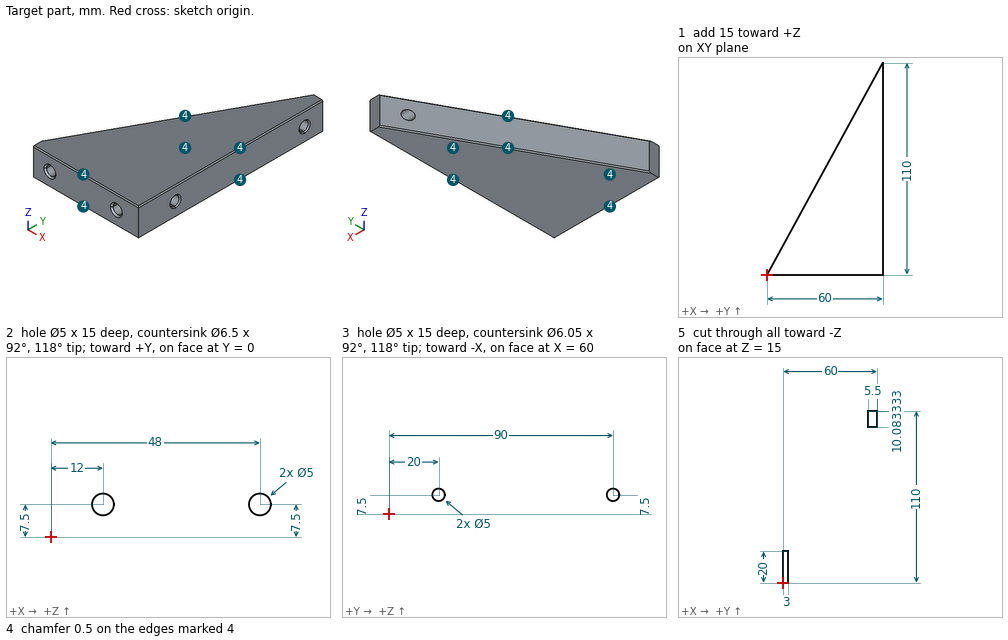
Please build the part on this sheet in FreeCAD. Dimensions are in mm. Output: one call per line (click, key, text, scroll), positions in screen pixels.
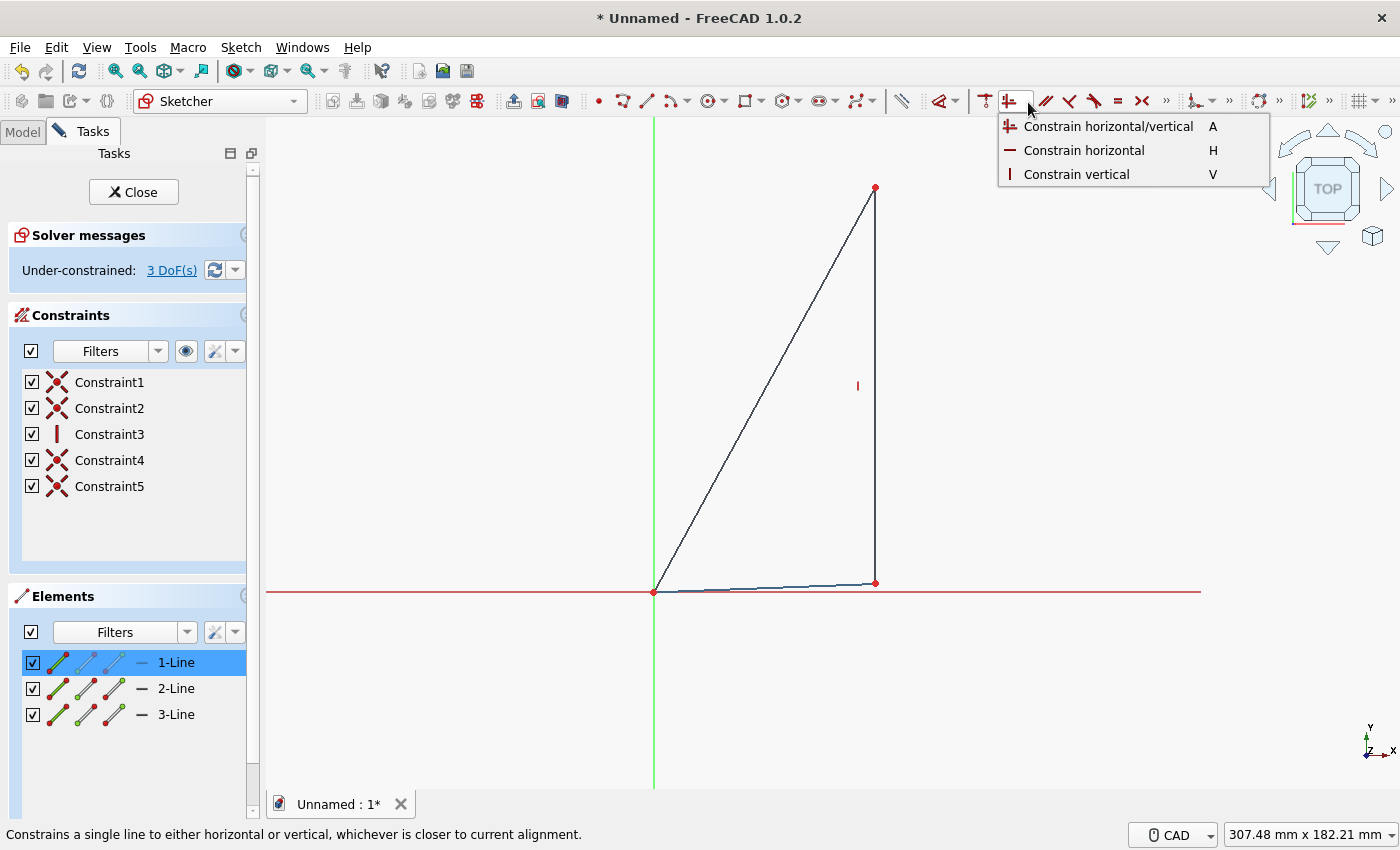
click(1134, 150)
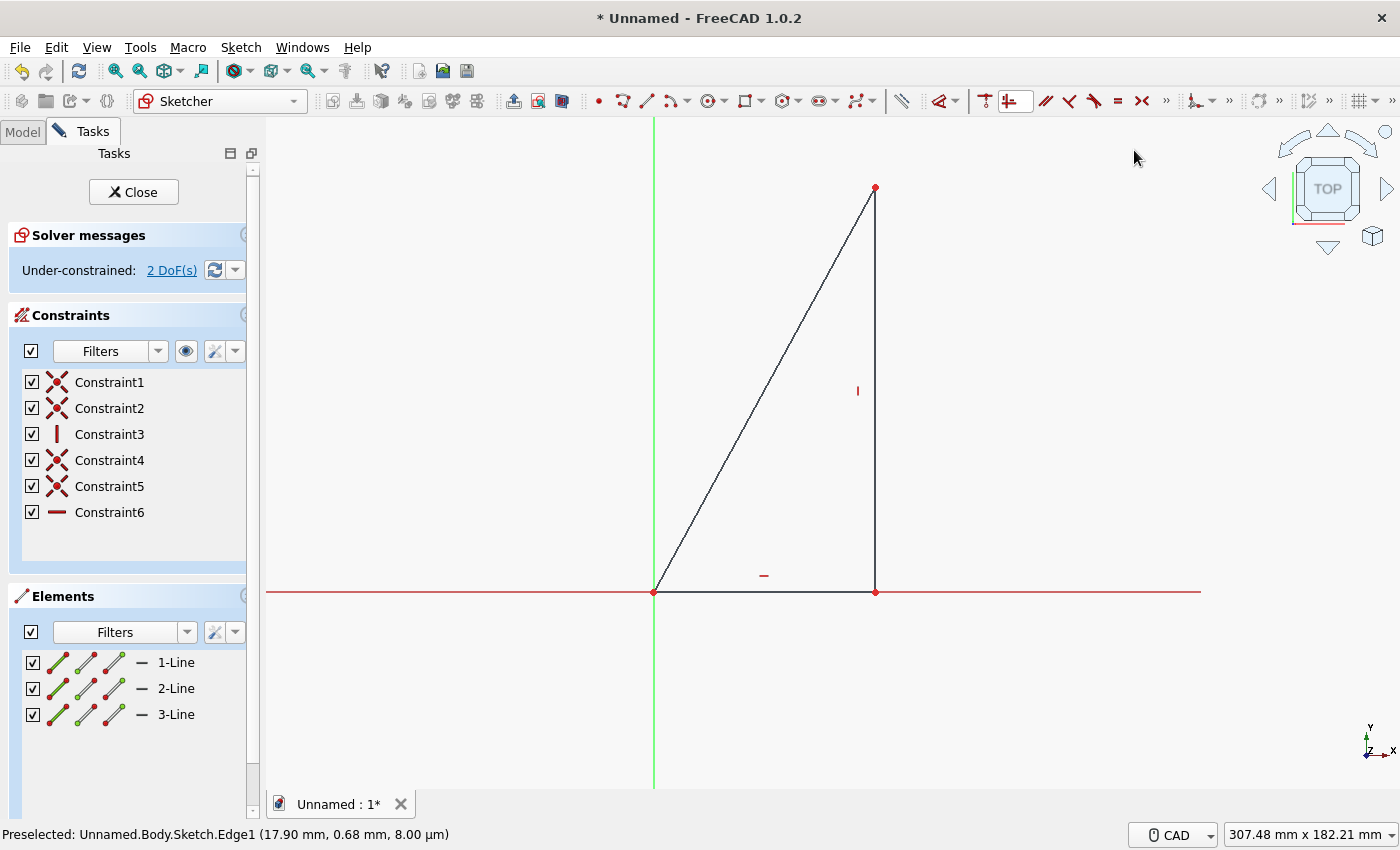
click(940, 102)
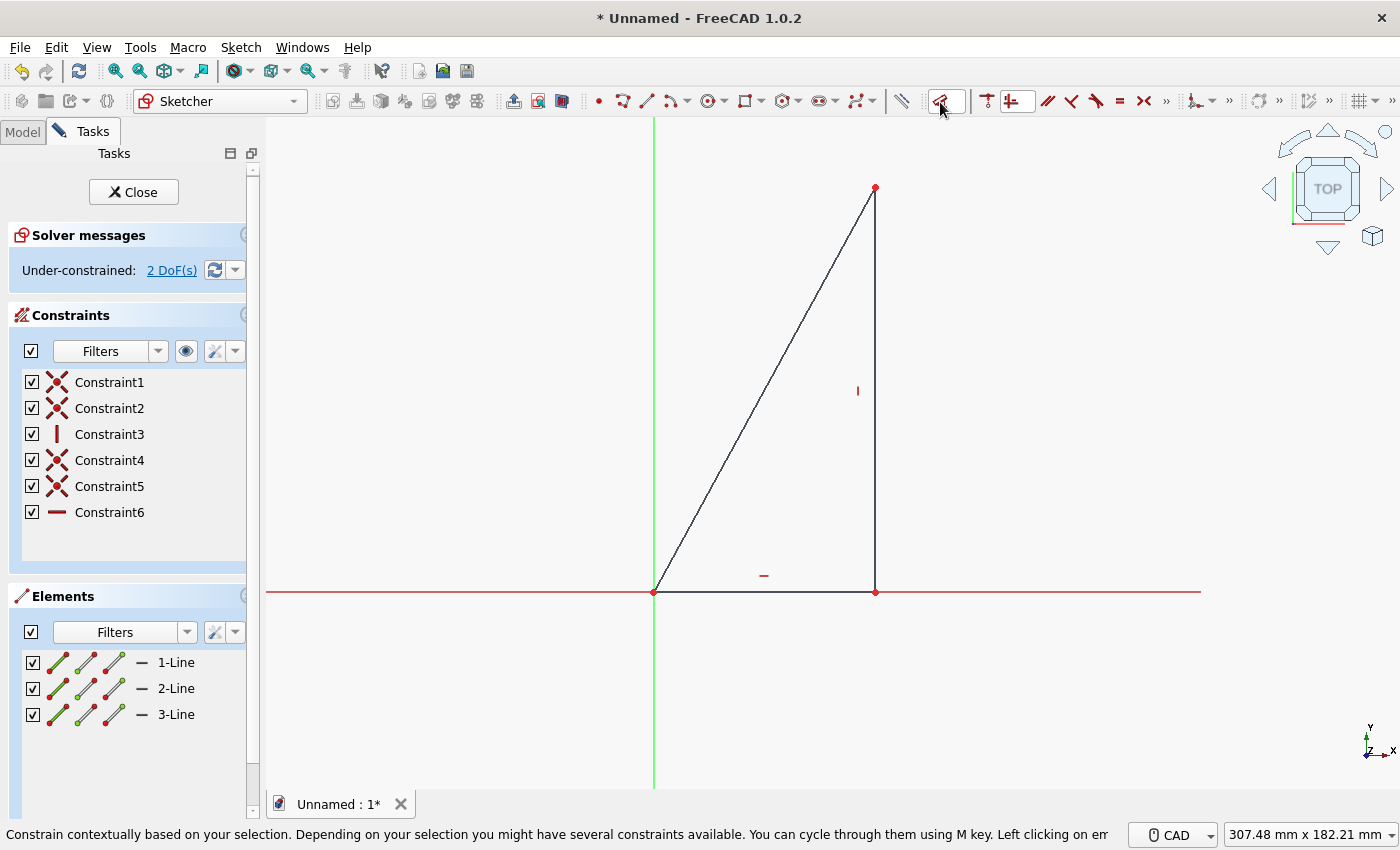
click(720, 592)
click(764, 626)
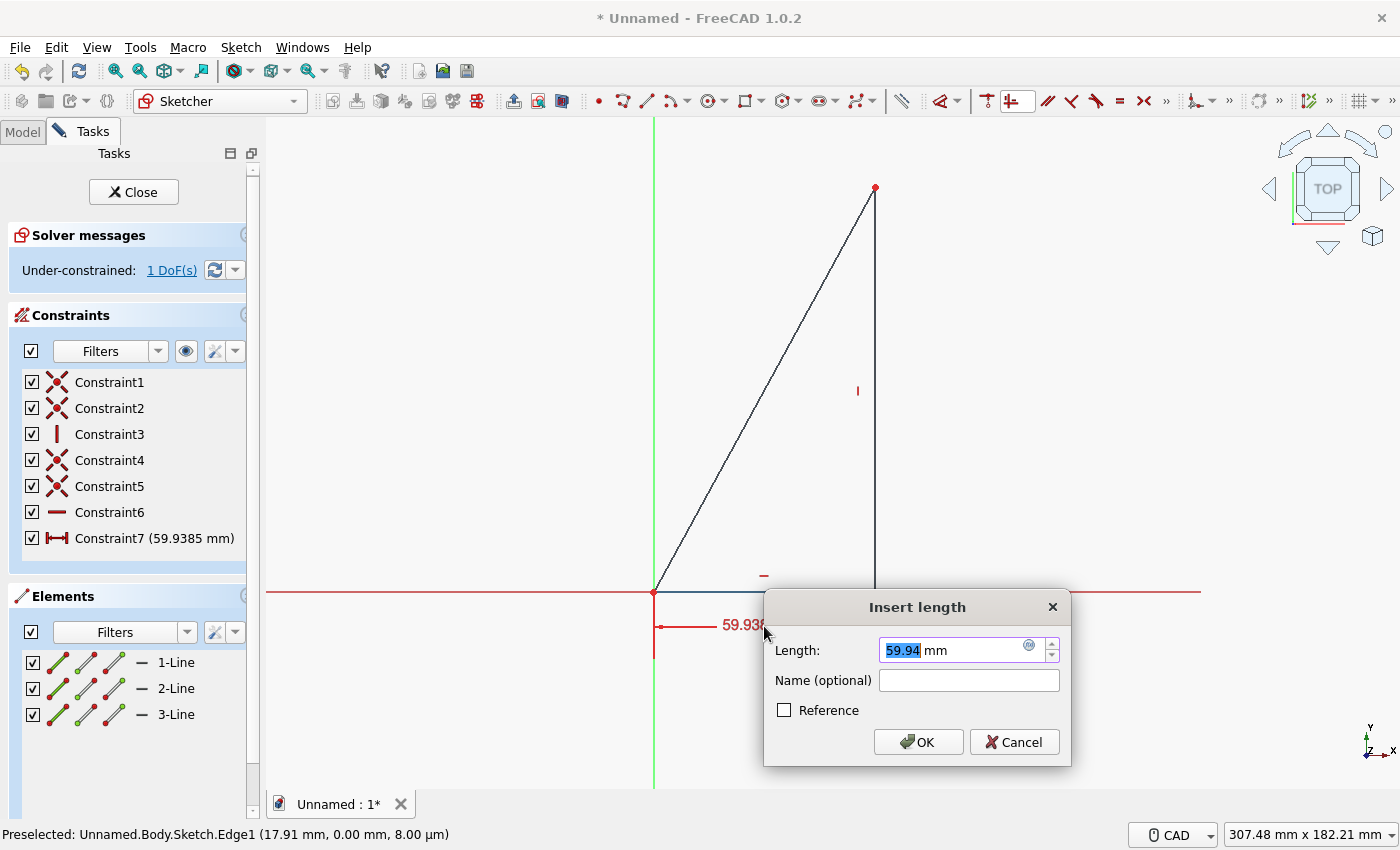
text(60)
key(Return)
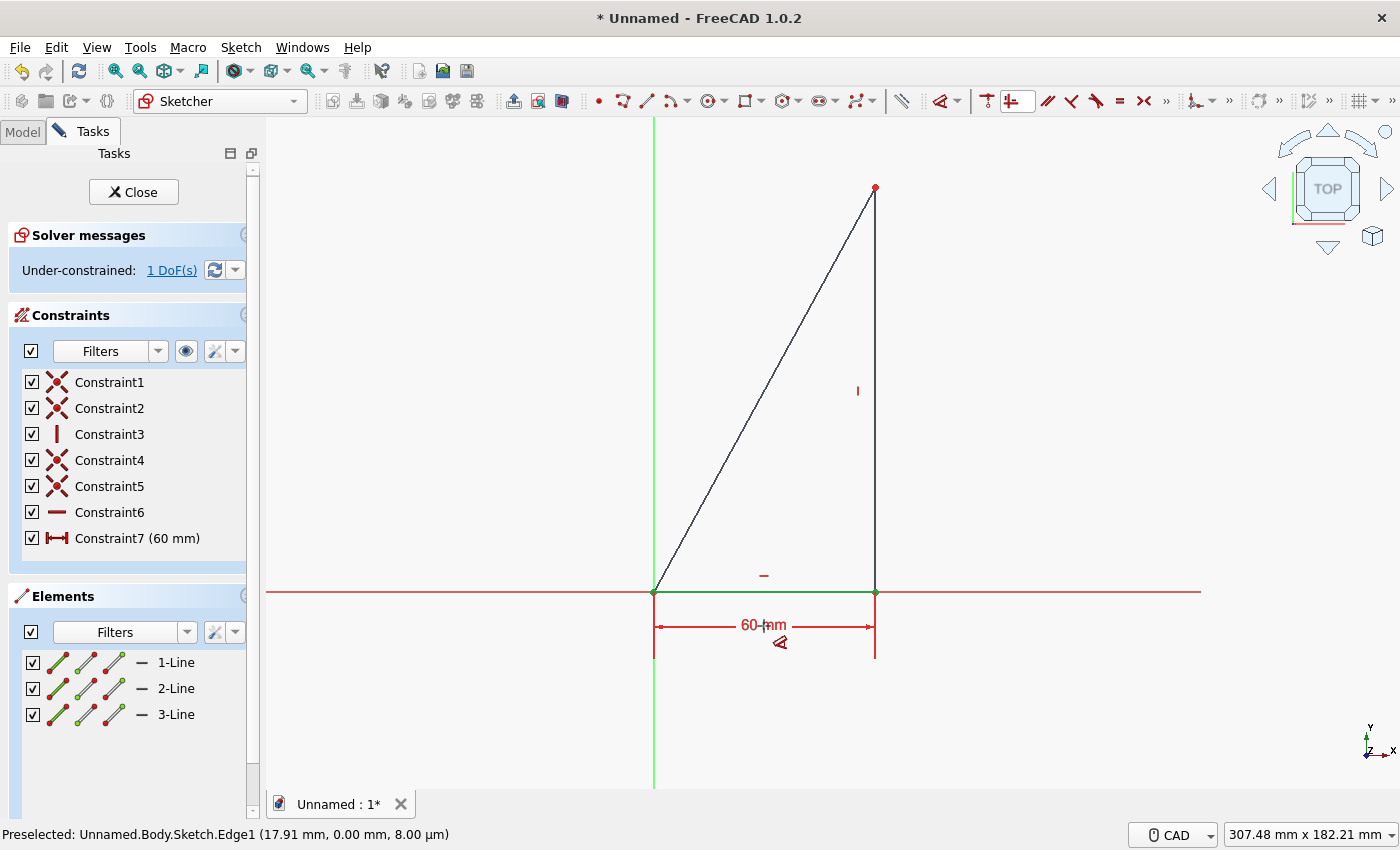
click(875, 471)
click(909, 390)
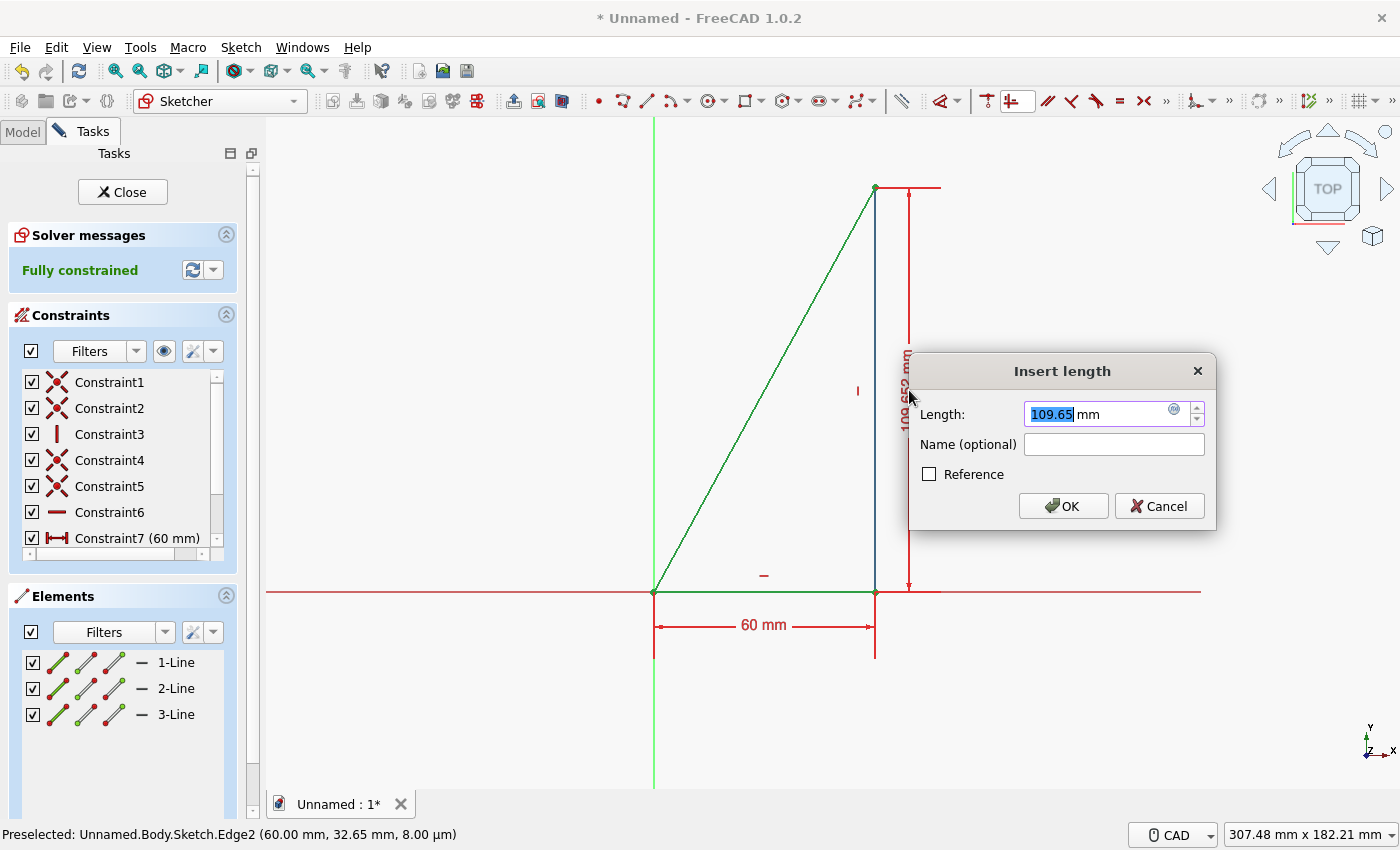
text(110)
key(Return)
key(Escape)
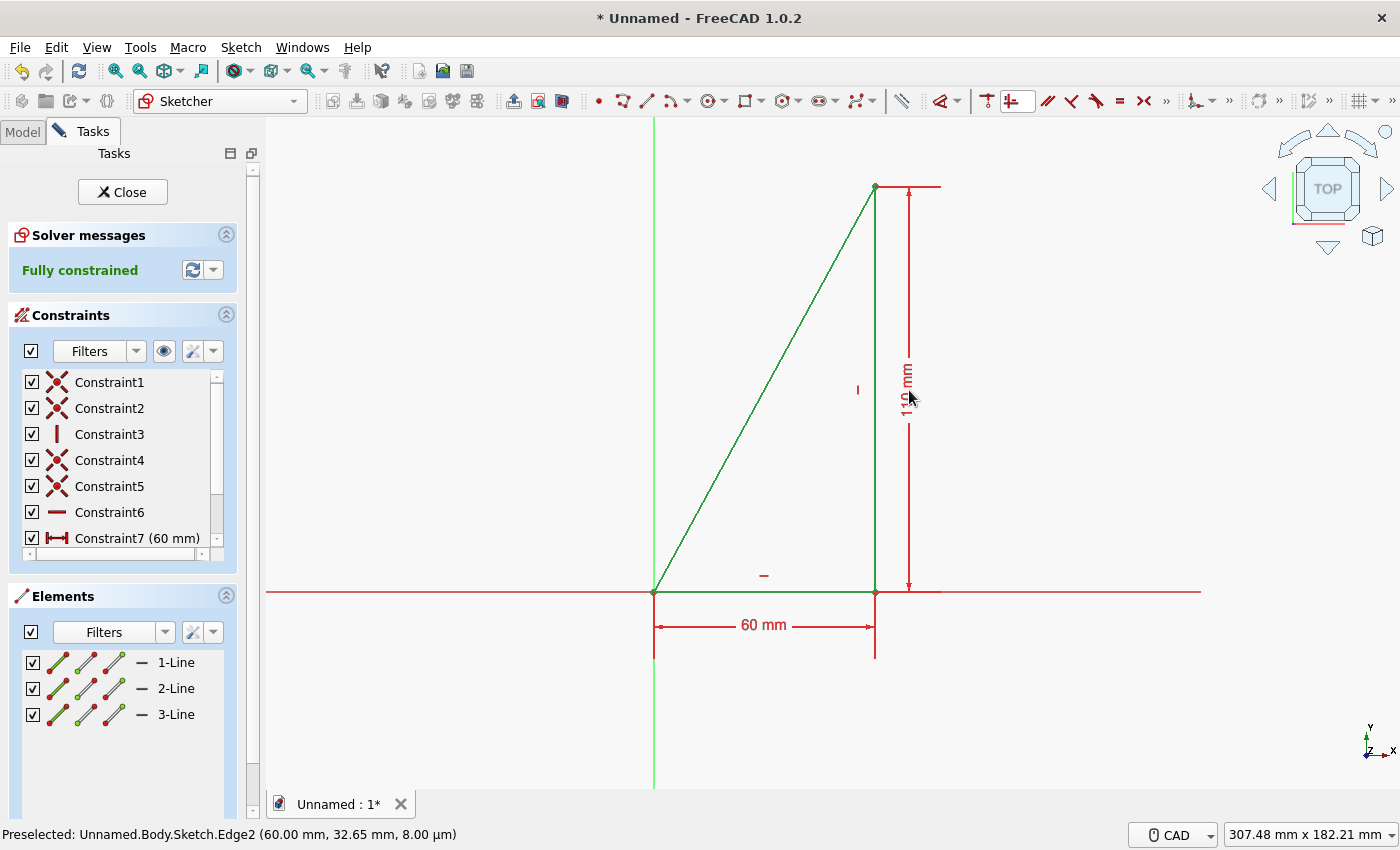
click(123, 192)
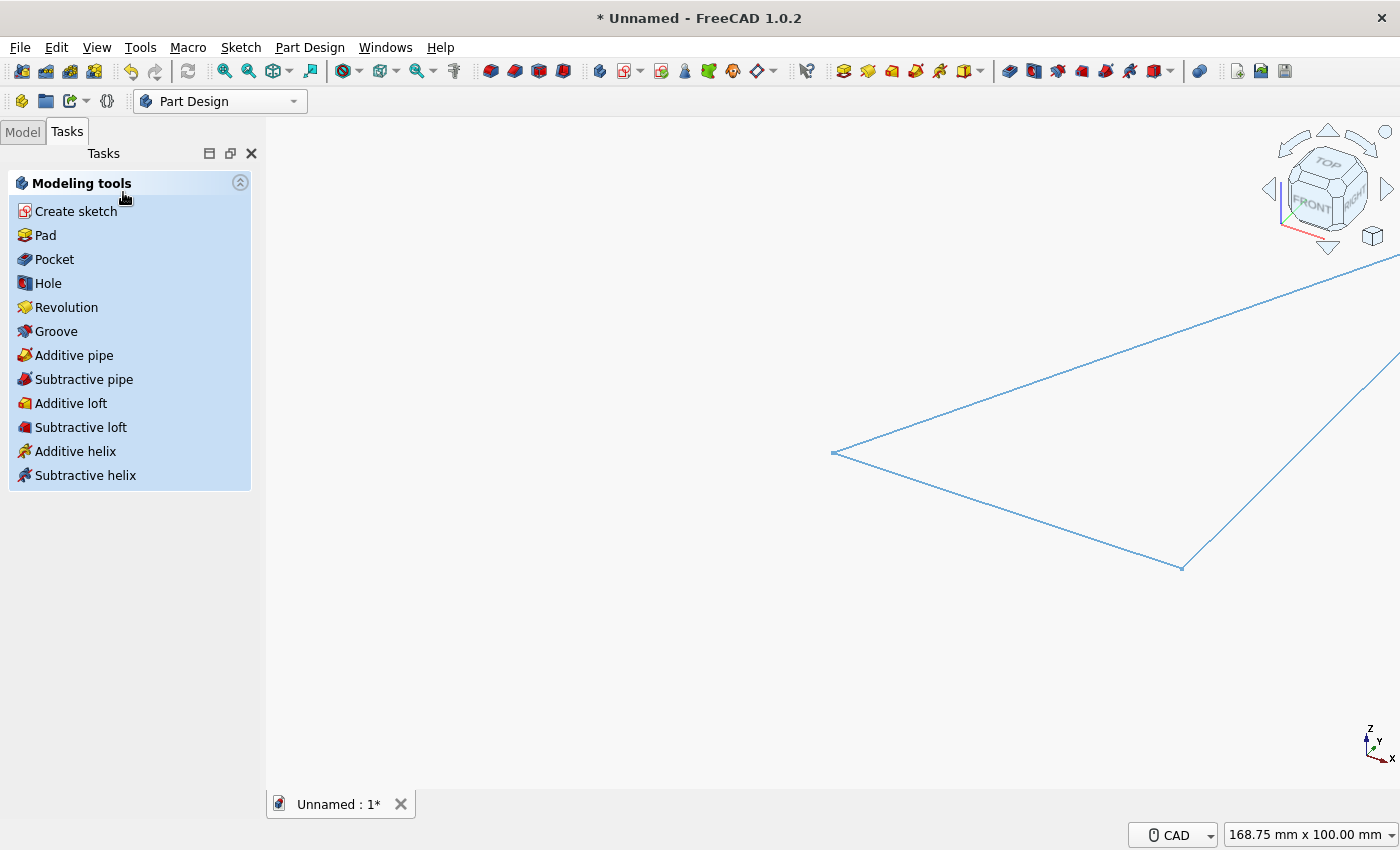
click(844, 72)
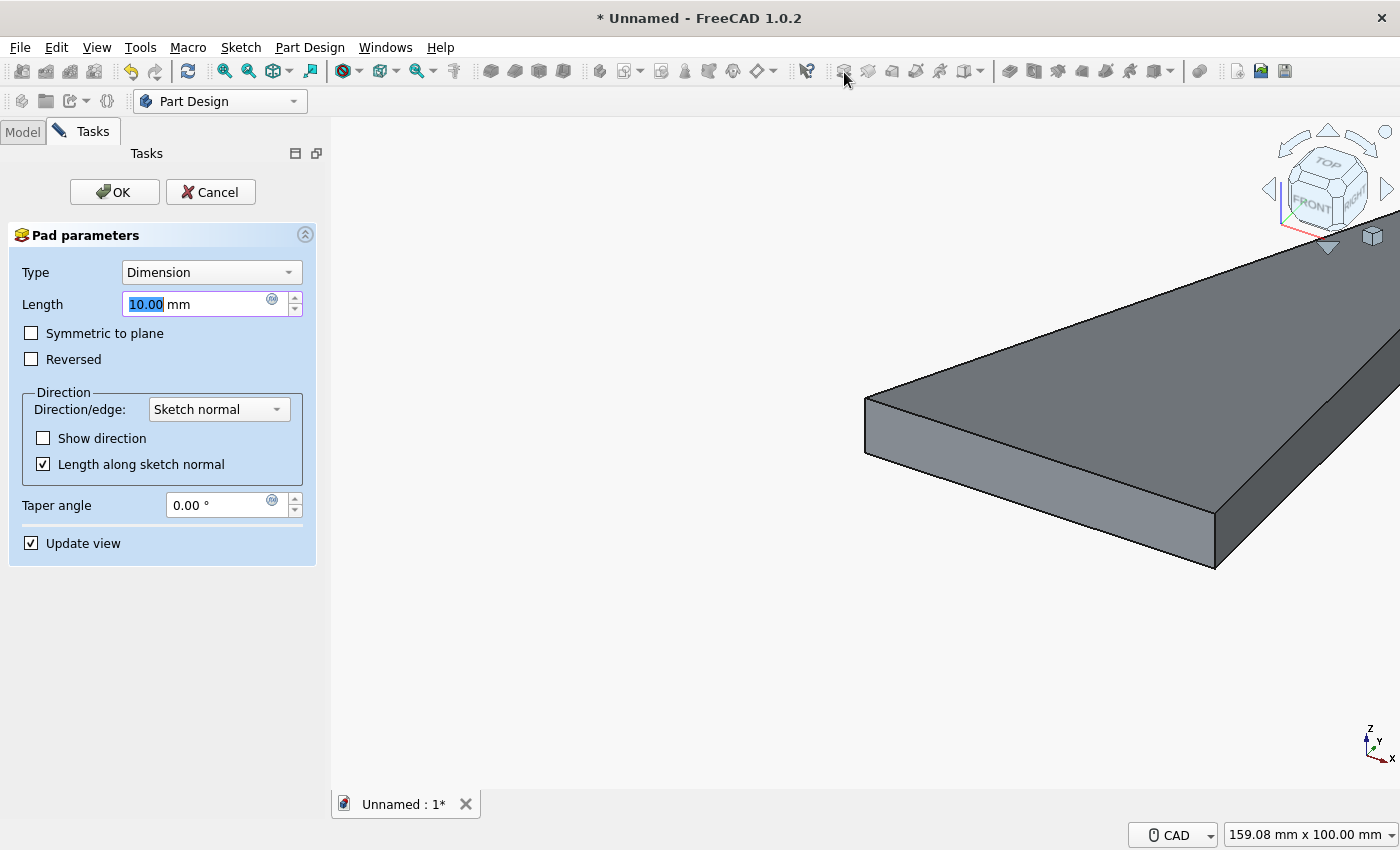
text(15)
key(Tab)